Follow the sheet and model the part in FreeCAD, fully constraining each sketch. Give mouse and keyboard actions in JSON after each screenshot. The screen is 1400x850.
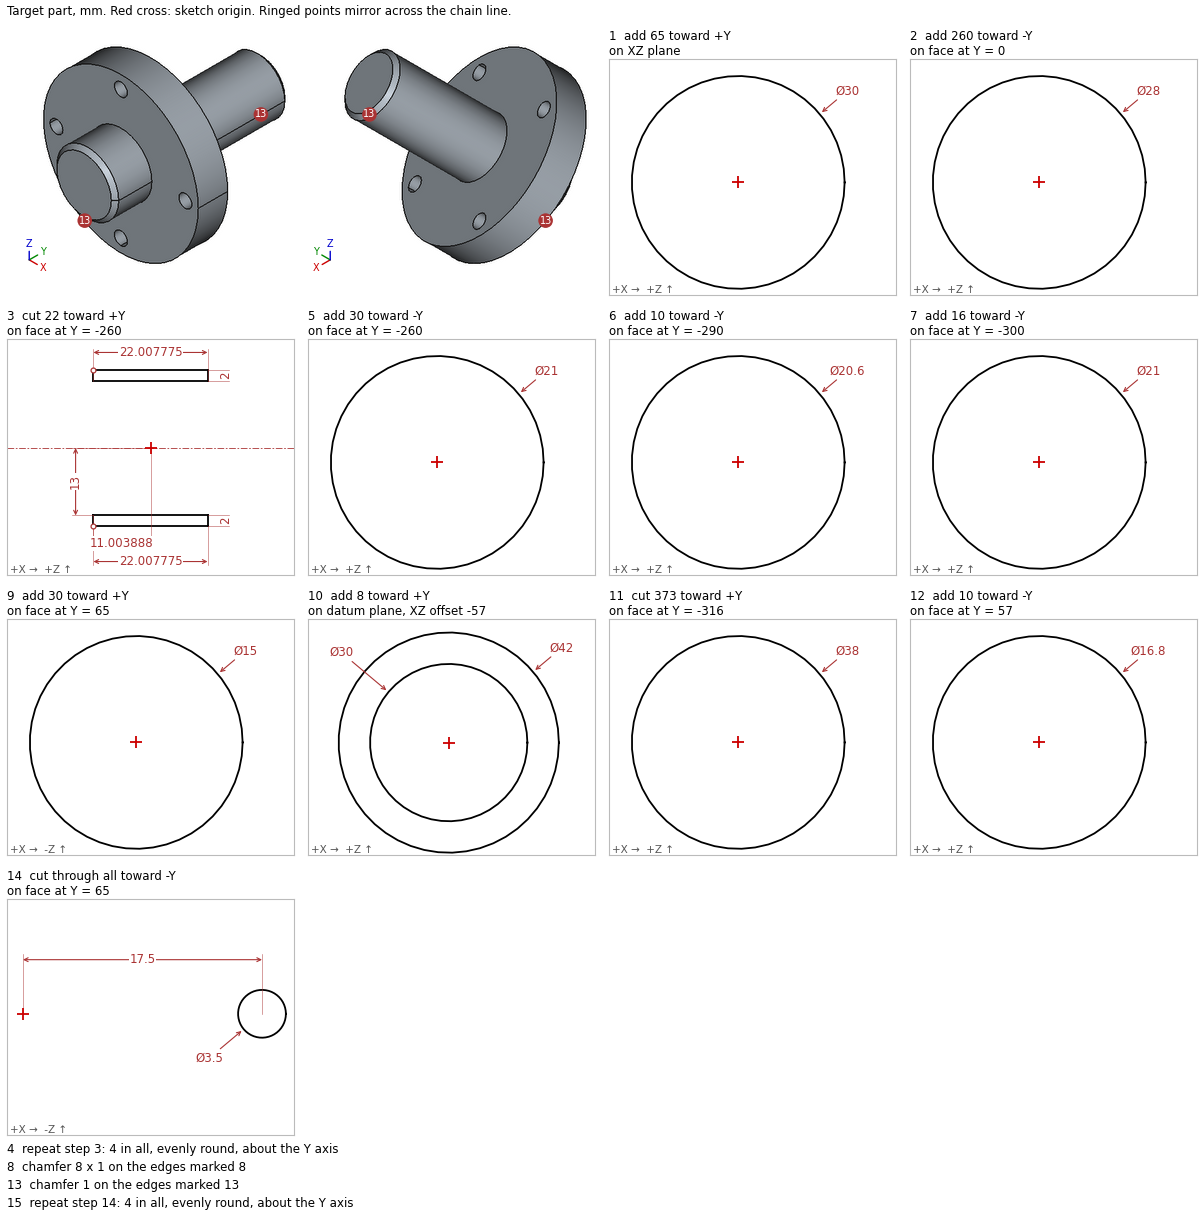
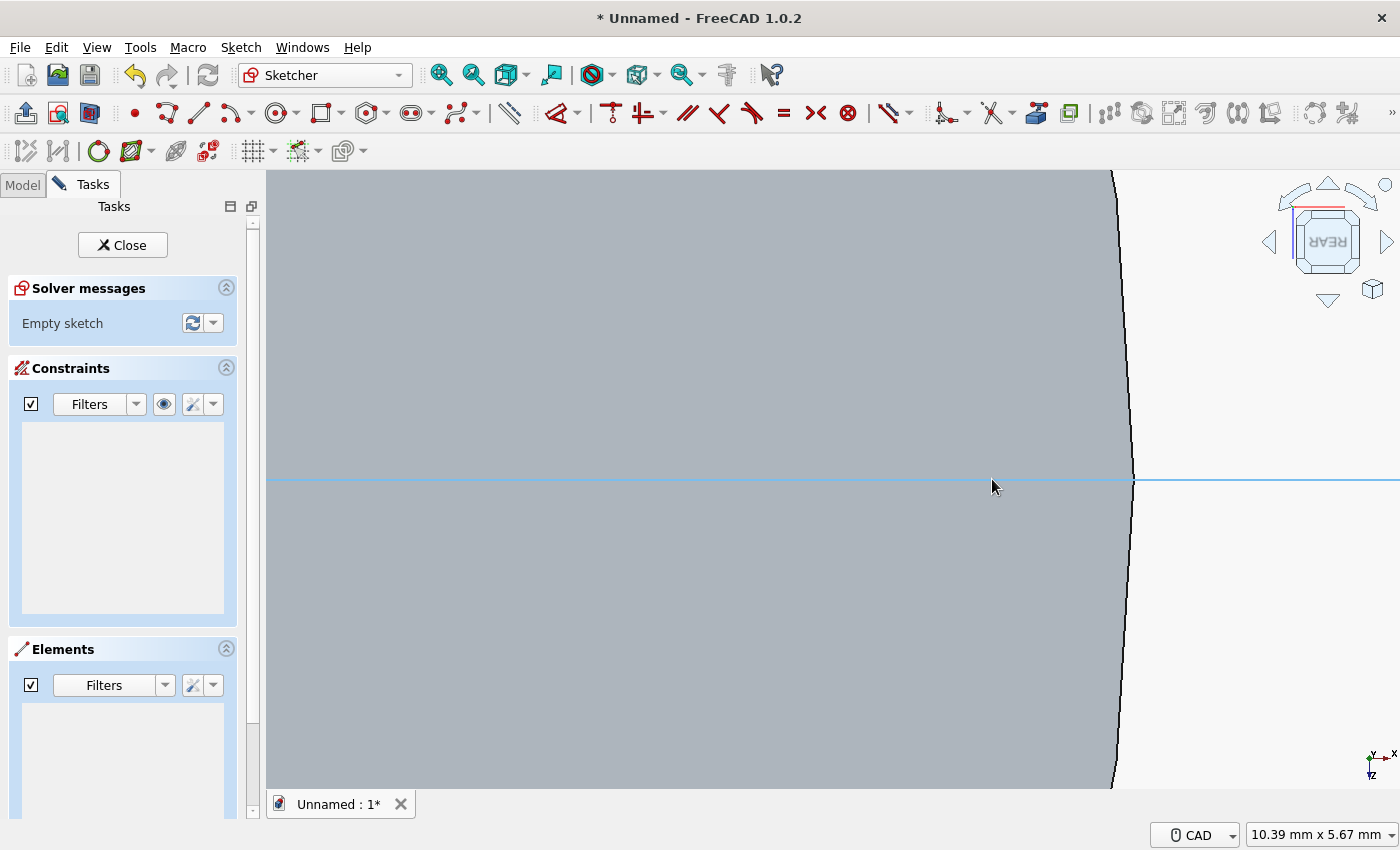
{"action": "left_click", "coordinate": [276, 114]}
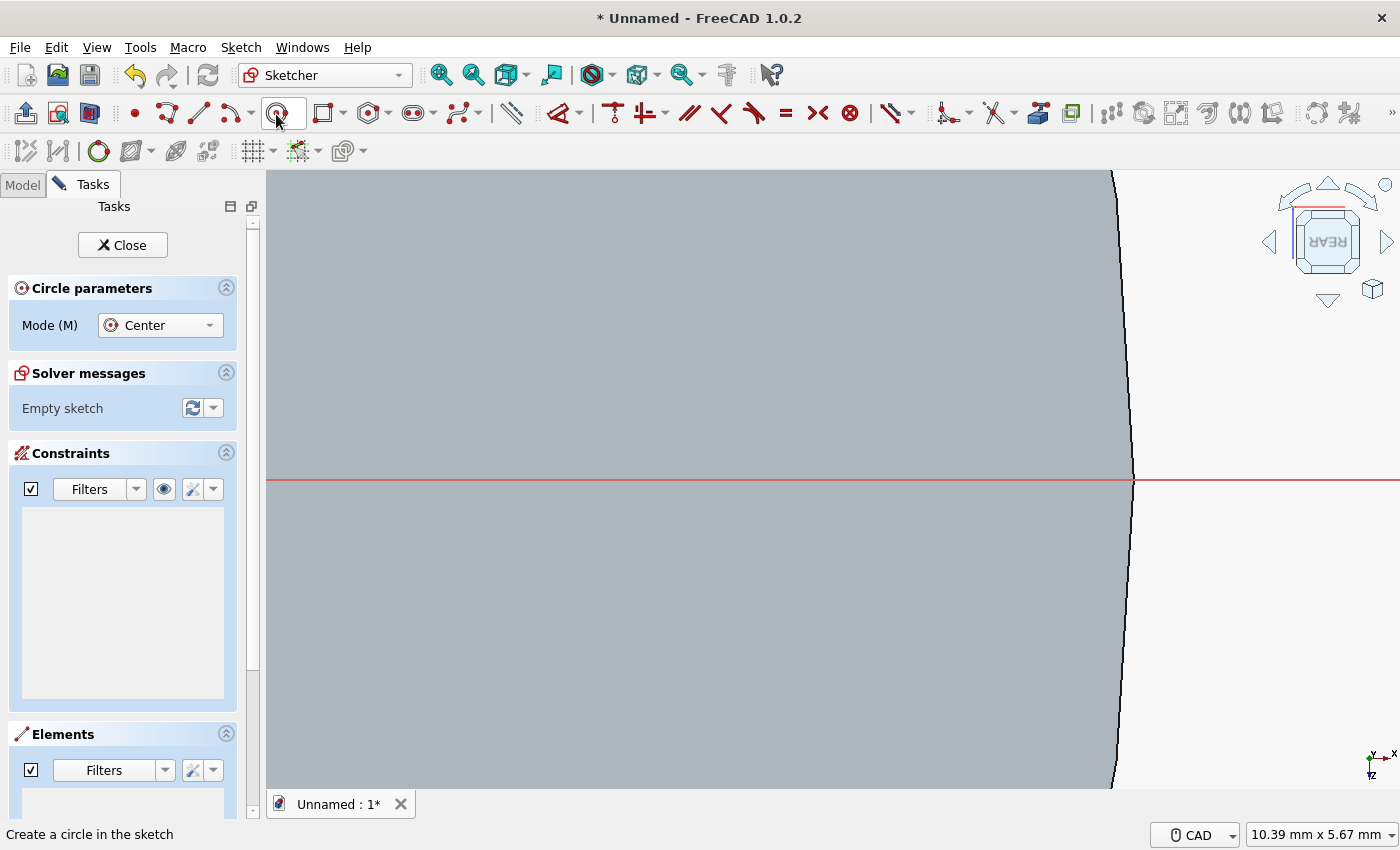
{"action": "left_click", "coordinate": [752, 479]}
{"action": "mouse_move", "coordinate": [887, 344]}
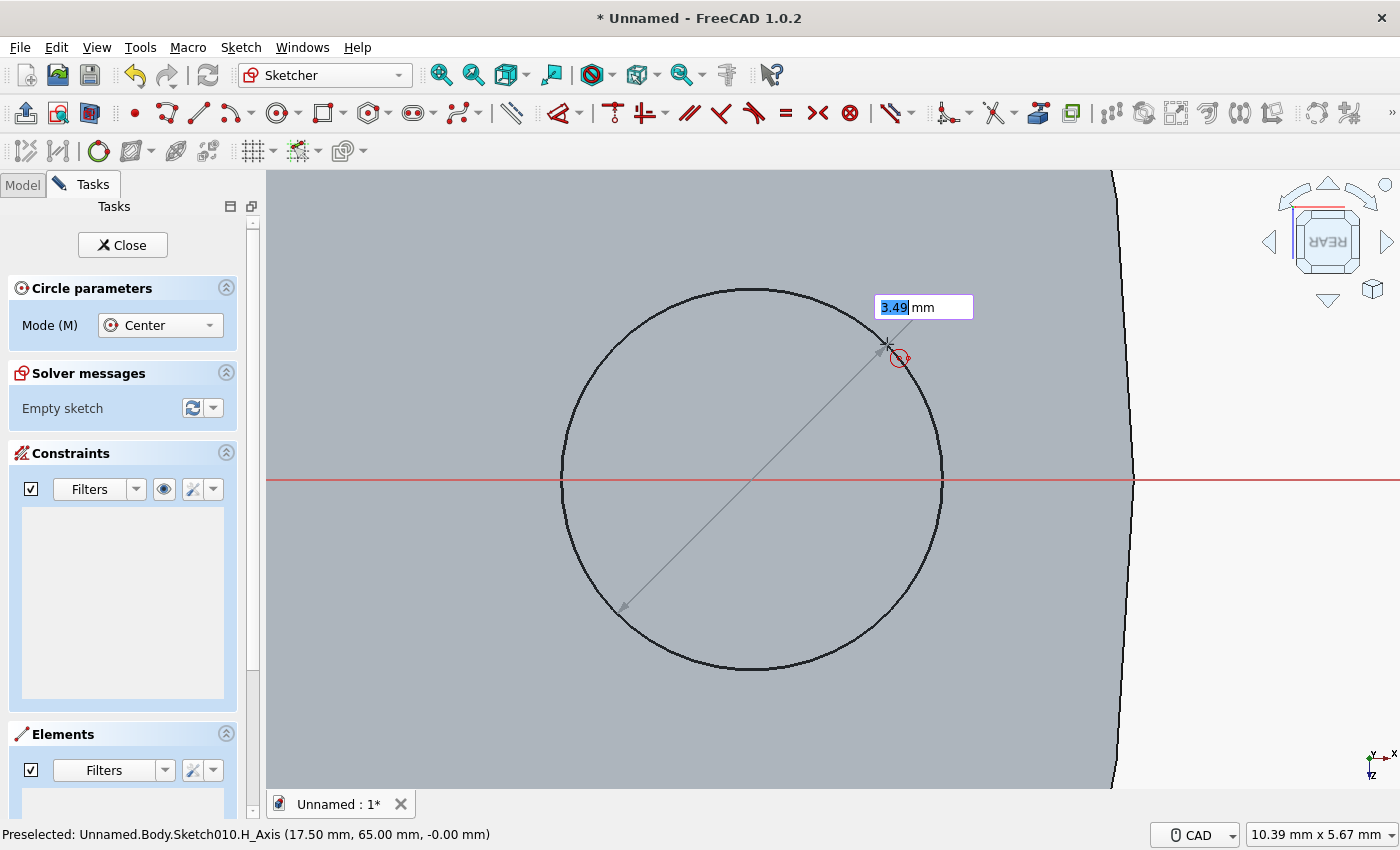
{"action": "type", "text": "3.5"}
{"action": "key", "text": "Return"}
{"action": "key", "text": "Escape"}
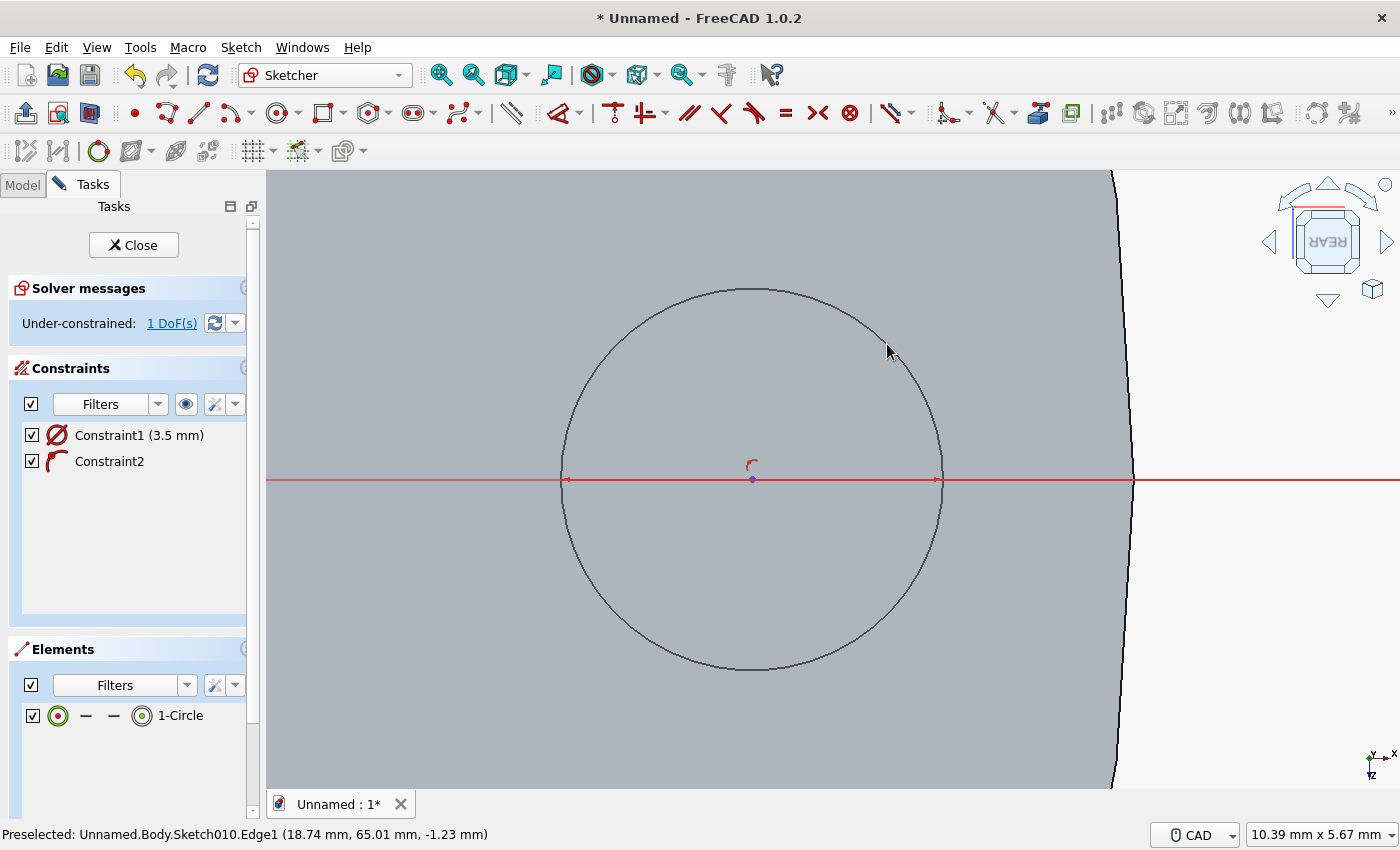
{"action": "key", "text": "d"}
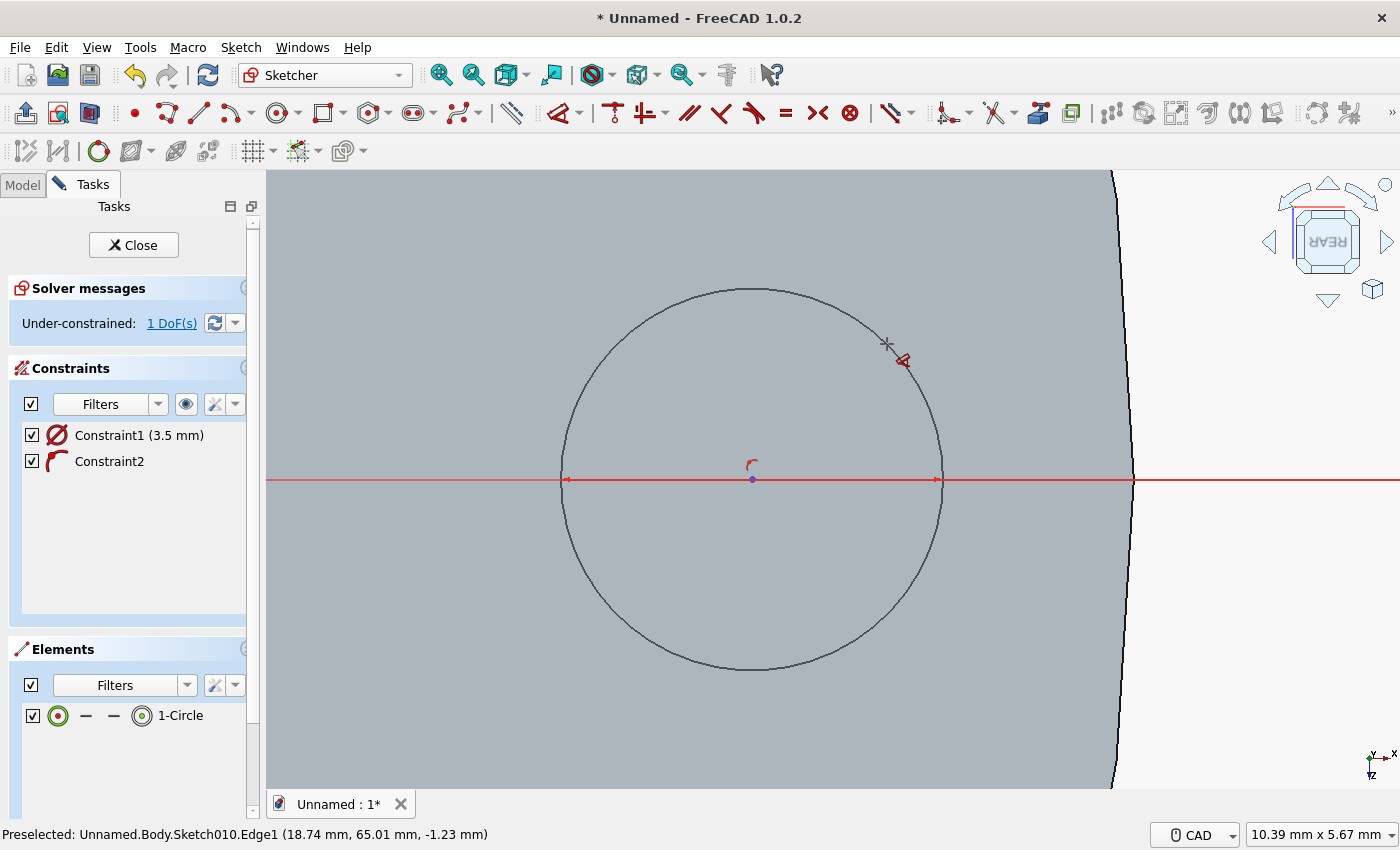
{"action": "left_click", "coordinate": [752, 479]}
{"action": "left_click", "coordinate": [523, 513]}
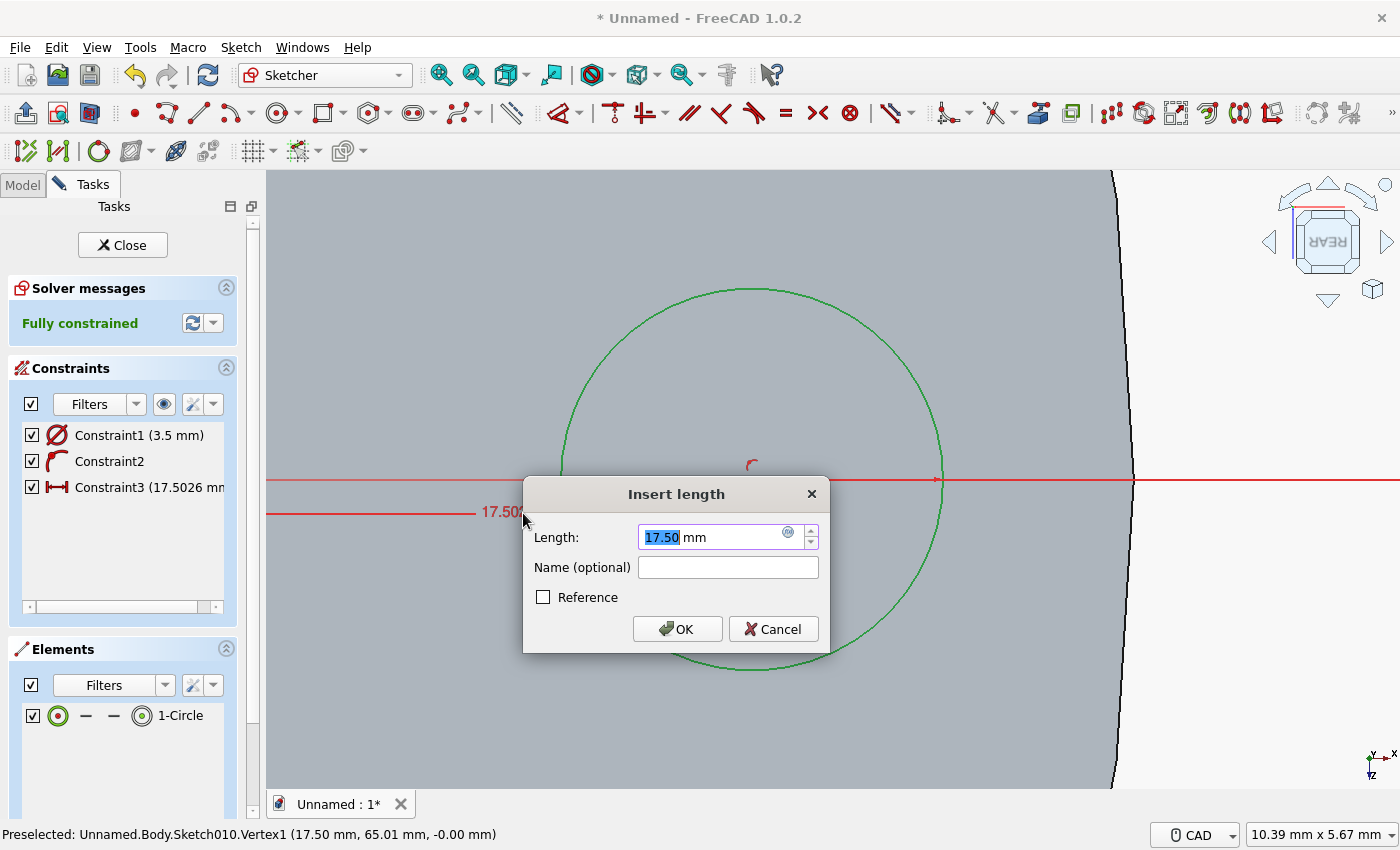
{"action": "type", "text": "17.5"}
{"action": "key", "text": "Return"}
{"action": "key", "text": "Escape"}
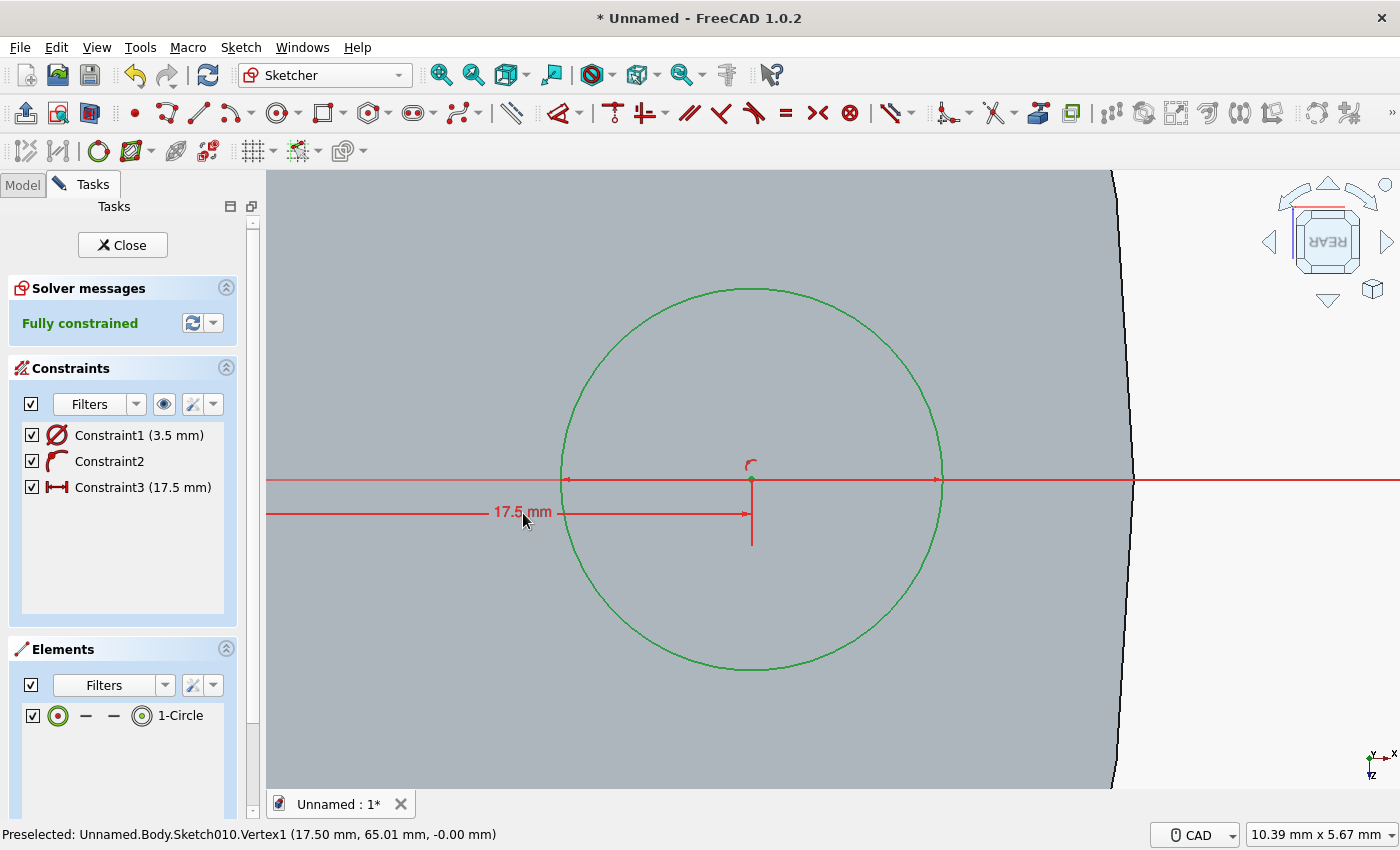
{"action": "left_click", "coordinate": [123, 245]}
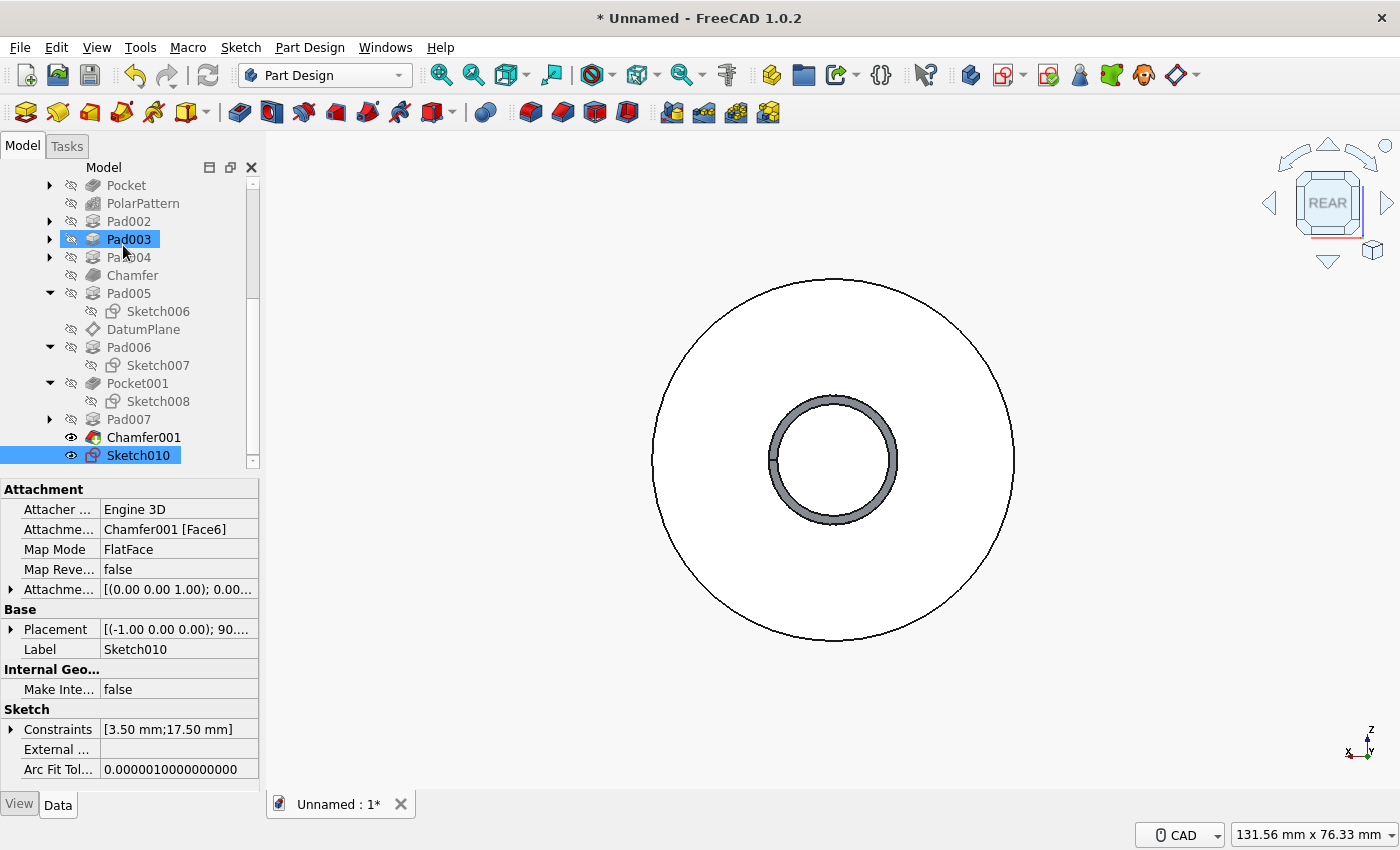
{"action": "left_click", "coordinate": [240, 112]}